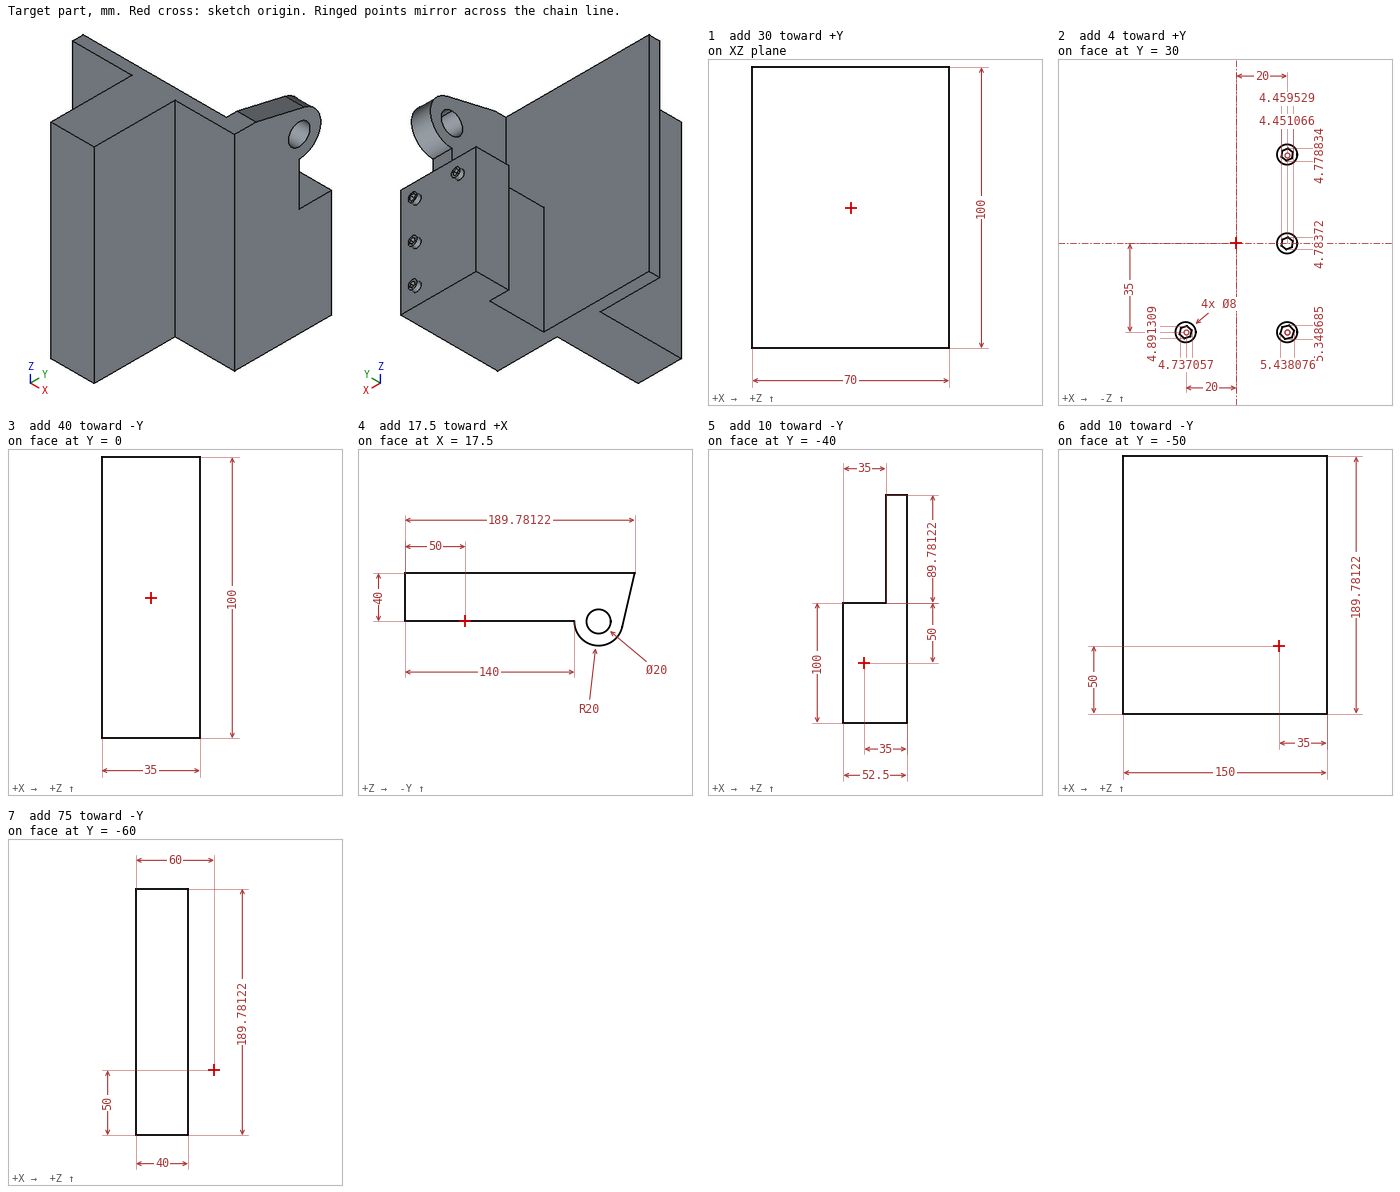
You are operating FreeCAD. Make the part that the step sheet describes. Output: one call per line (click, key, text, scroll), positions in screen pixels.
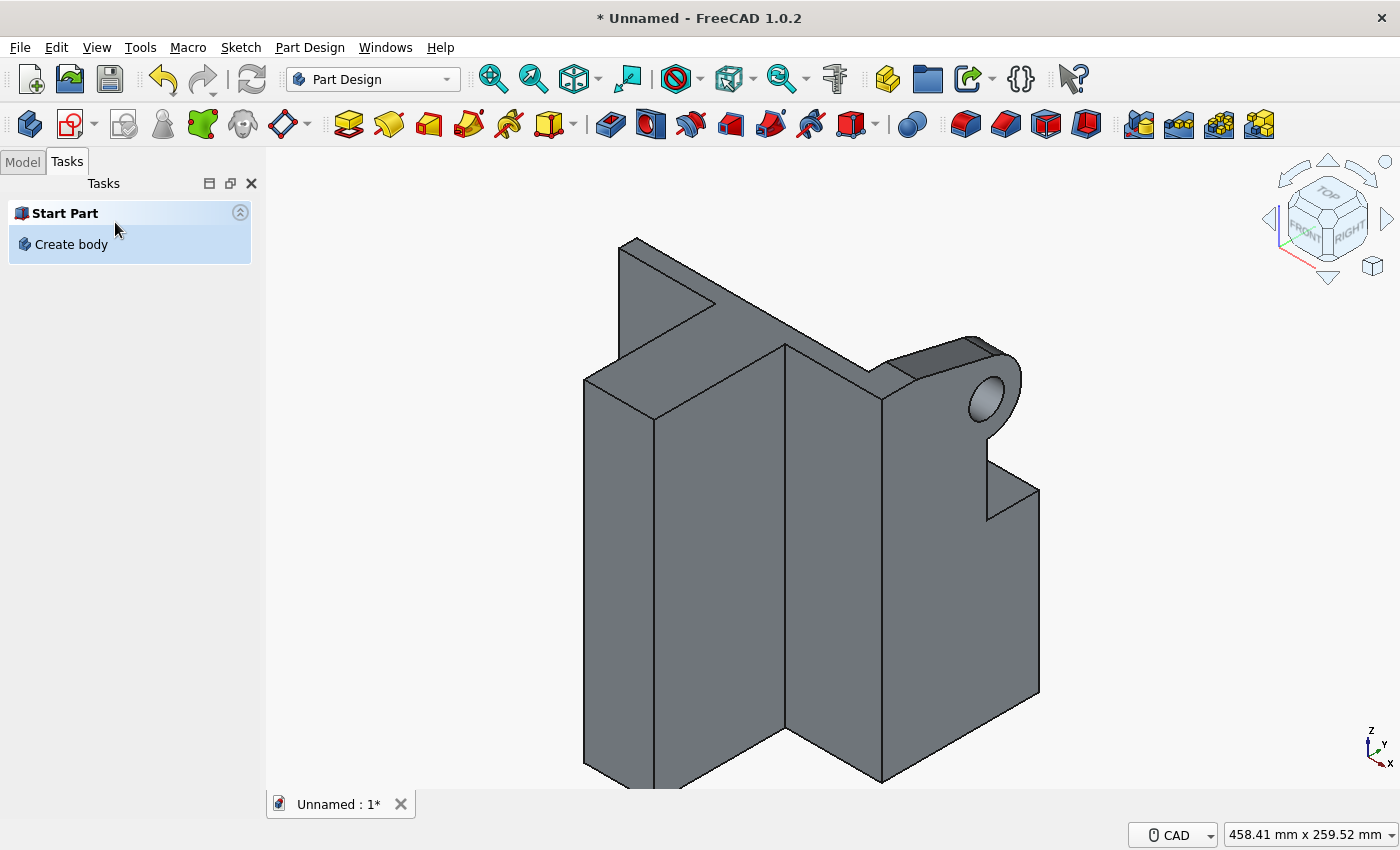
click(494, 80)